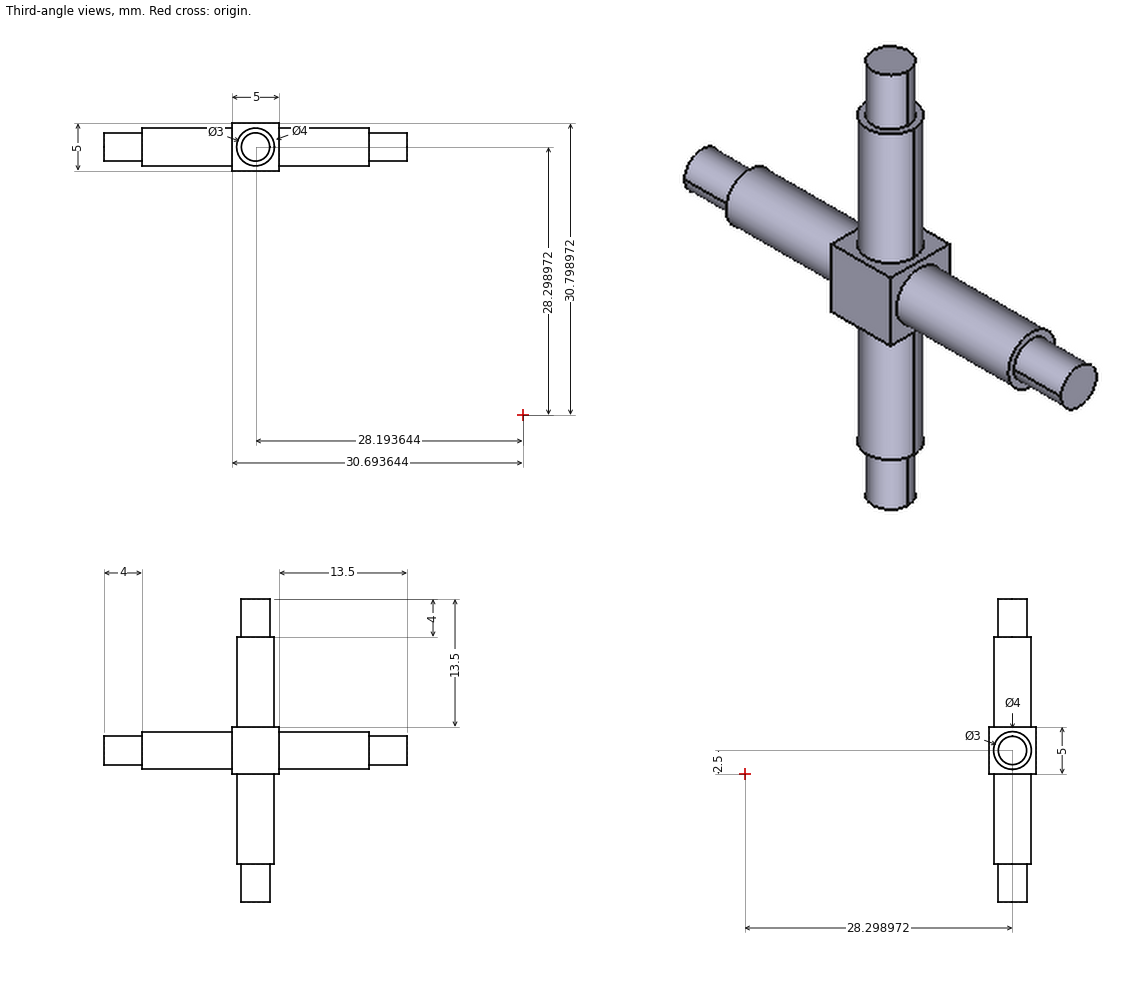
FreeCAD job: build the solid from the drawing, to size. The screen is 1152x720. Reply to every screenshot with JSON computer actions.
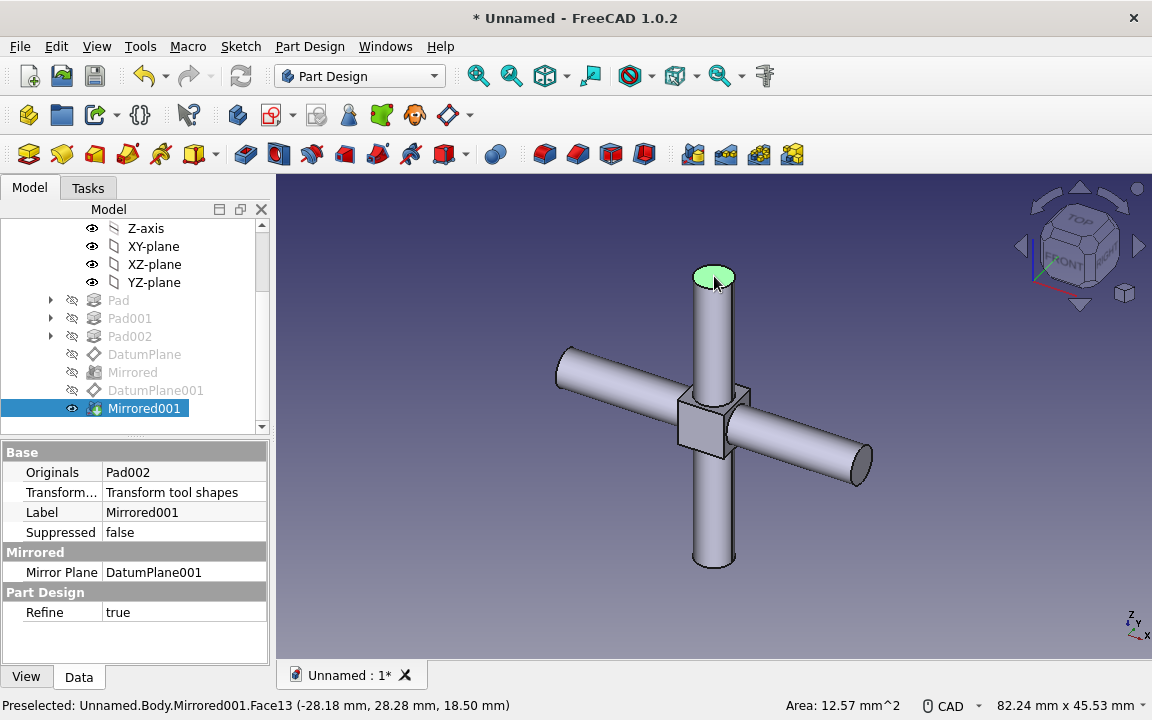
{"action": "left_click", "coordinate": [270, 116]}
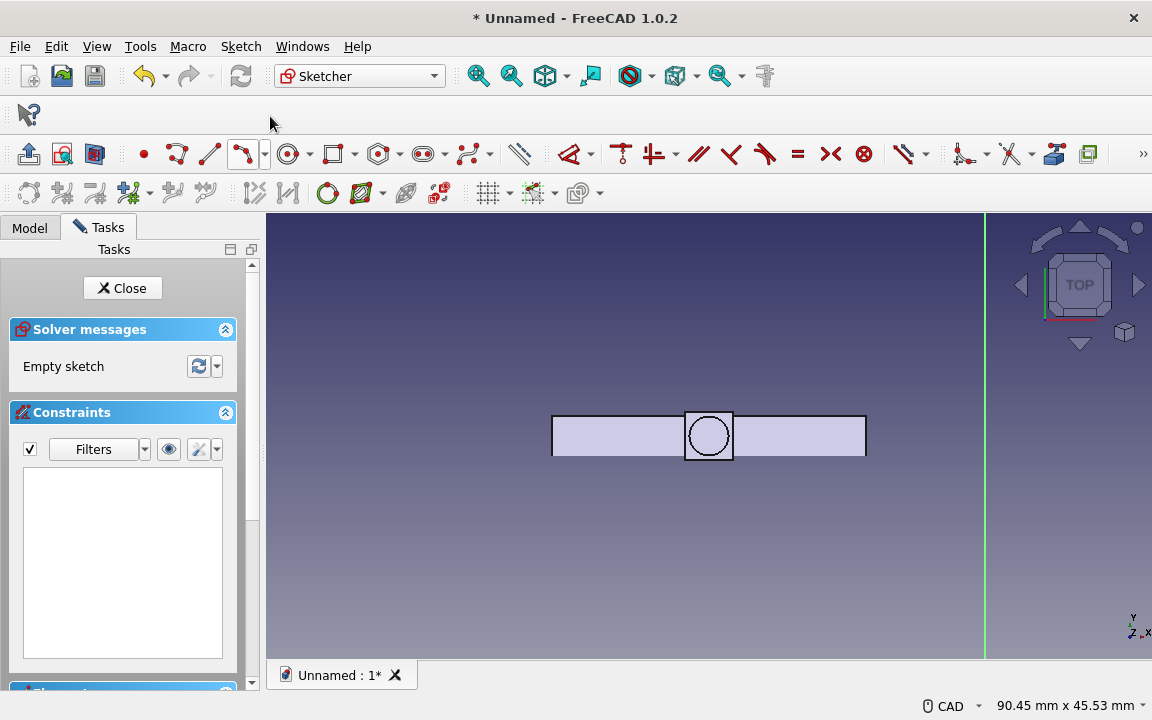
{"action": "scroll", "coordinate": [720, 436], "scroll_direction": "up", "scroll_amount": 10}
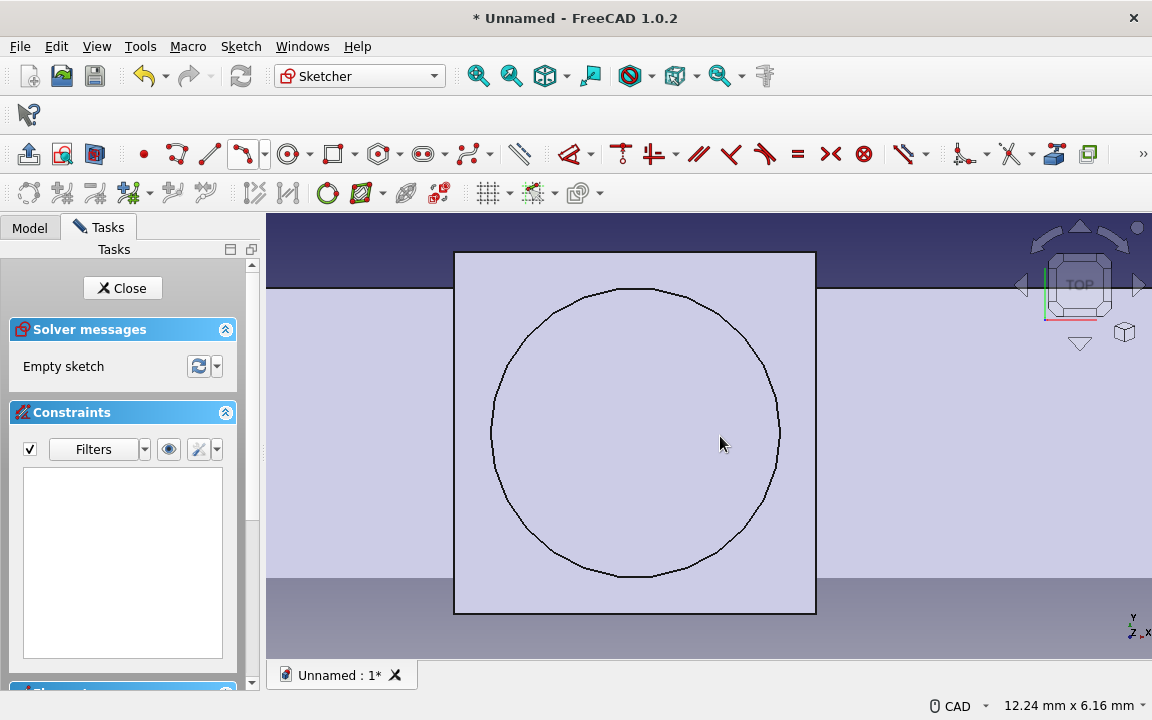
{"action": "key", "text": "g c"}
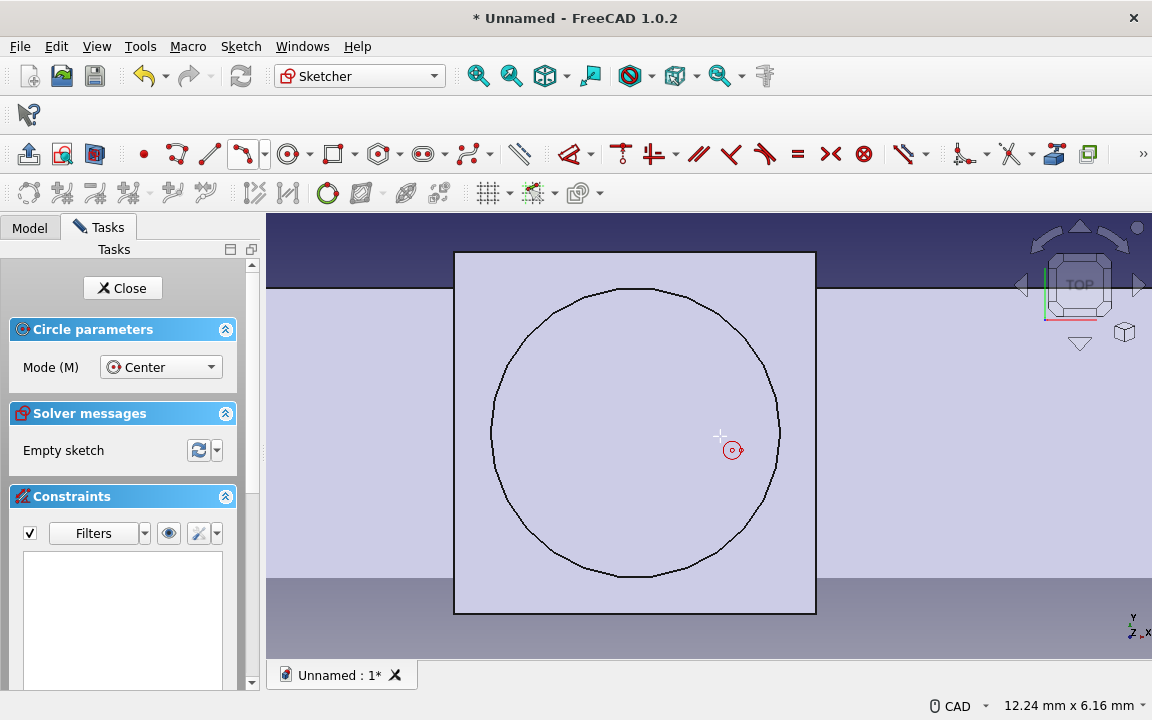
{"action": "left_click", "coordinate": [635, 433]}
{"action": "left_click", "coordinate": [738, 330]}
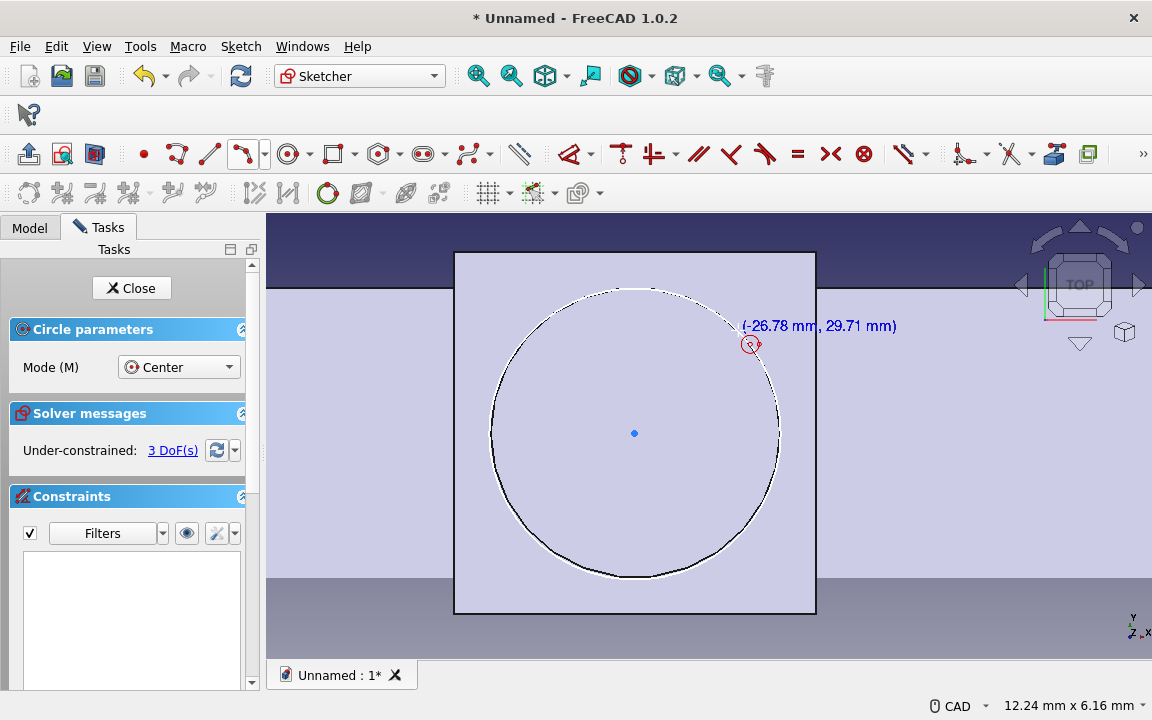
{"action": "left_click", "coordinate": [635, 434]}
{"action": "left_click", "coordinate": [712, 356]}
{"action": "key", "text": "Escape"}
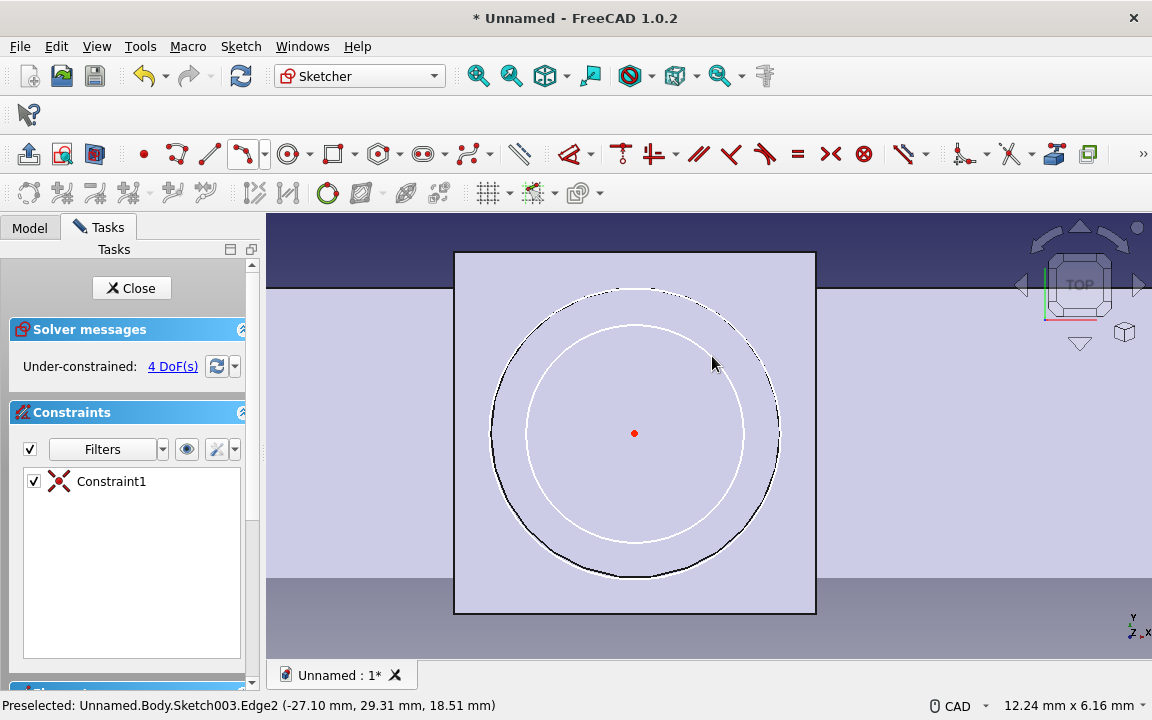
{"action": "left_click", "coordinate": [568, 154]}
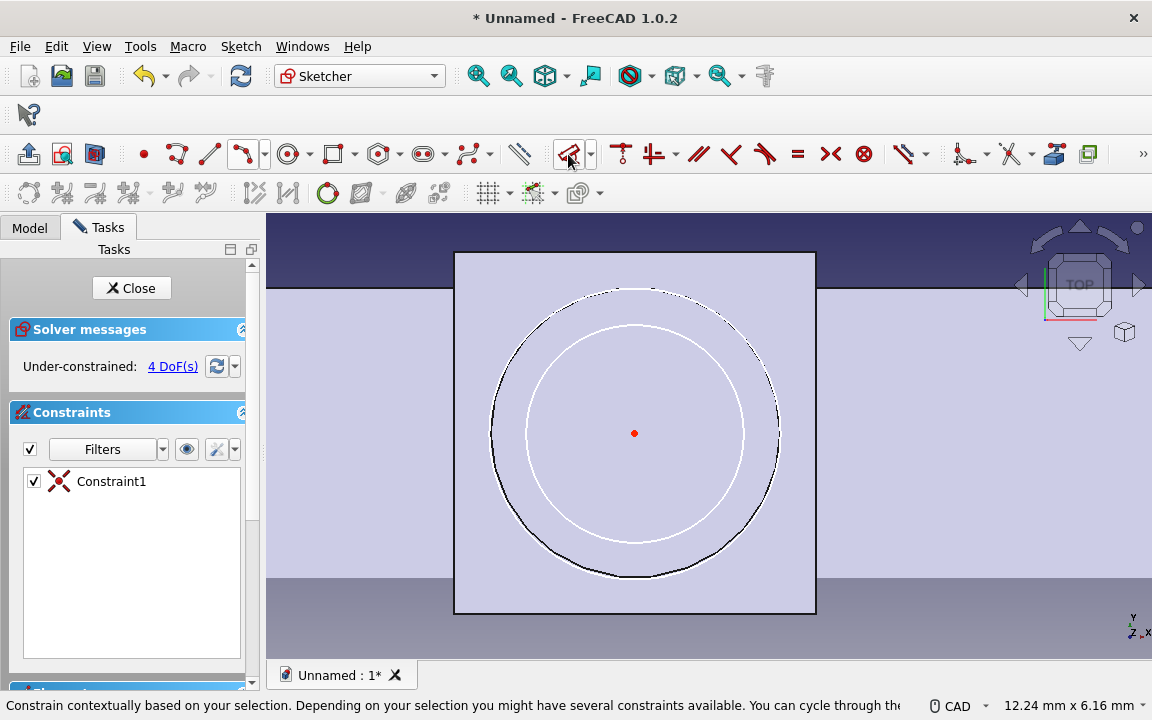
{"action": "left_click", "coordinate": [738, 331]}
{"action": "left_click", "coordinate": [761, 308]}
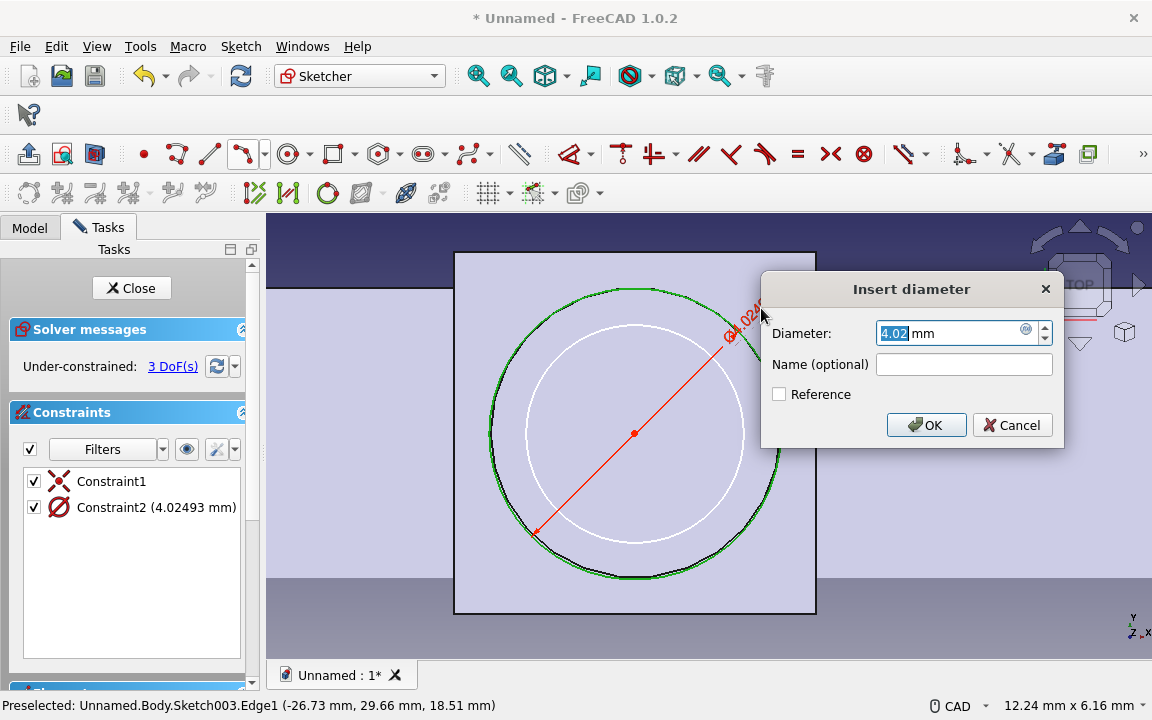
{"action": "type", "text": "4"}
{"action": "key", "text": "Return"}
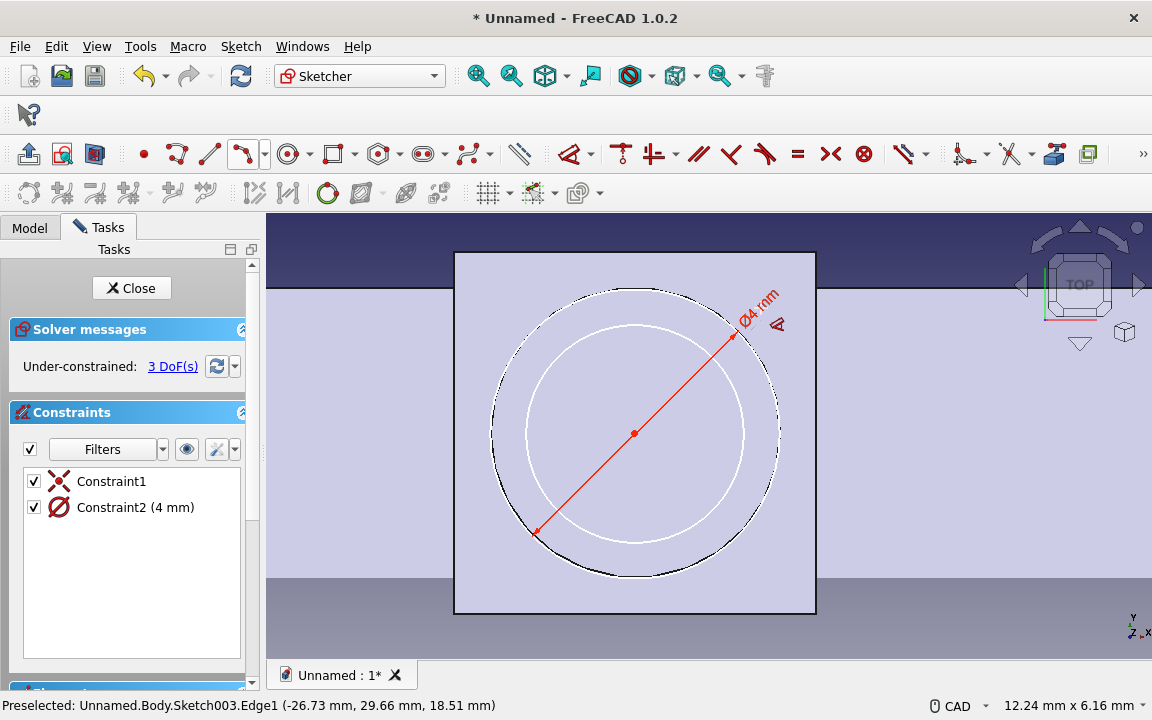
{"action": "left_click", "coordinate": [712, 357]}
{"action": "left_click", "coordinate": [792, 388]}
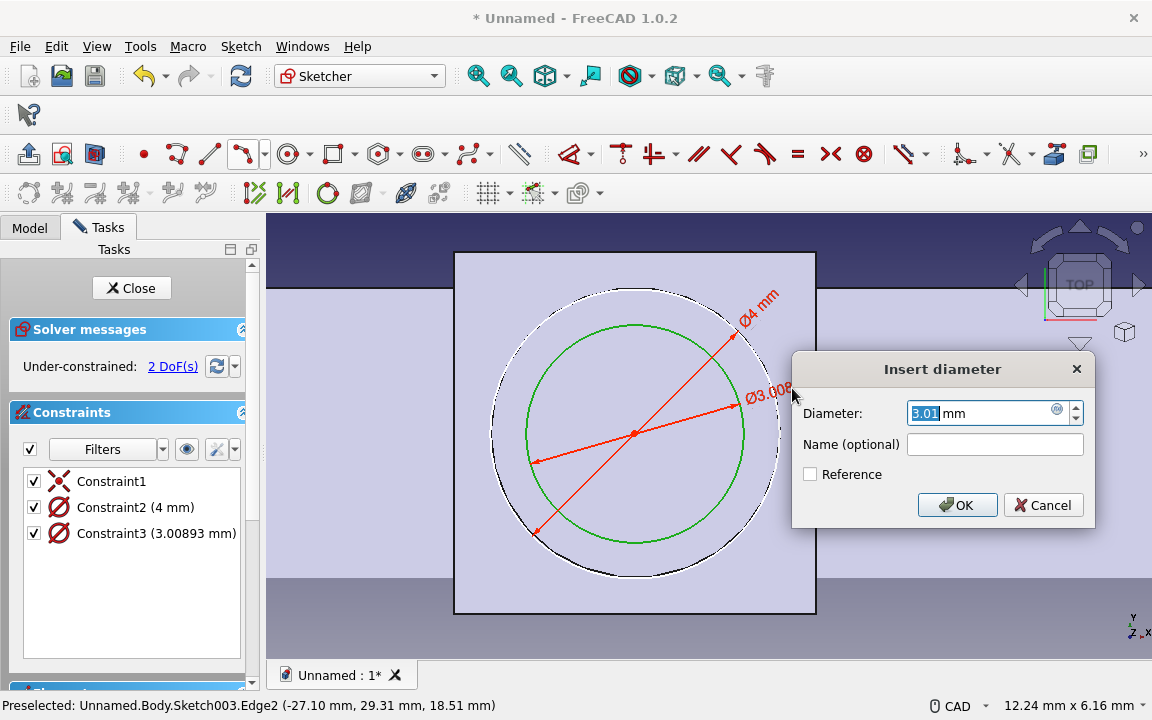
{"action": "type", "text": "3"}
{"action": "key", "text": "Return"}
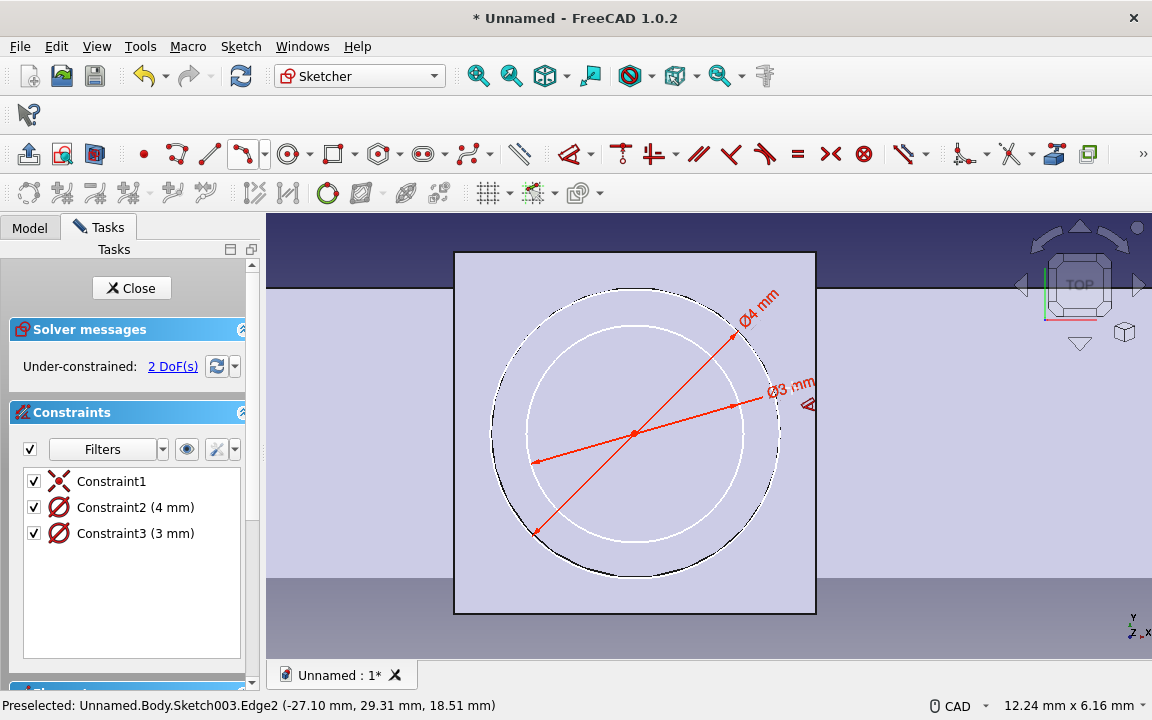
{"action": "left_click", "coordinate": [635, 434]}
{"action": "left_click", "coordinate": [892, 400]}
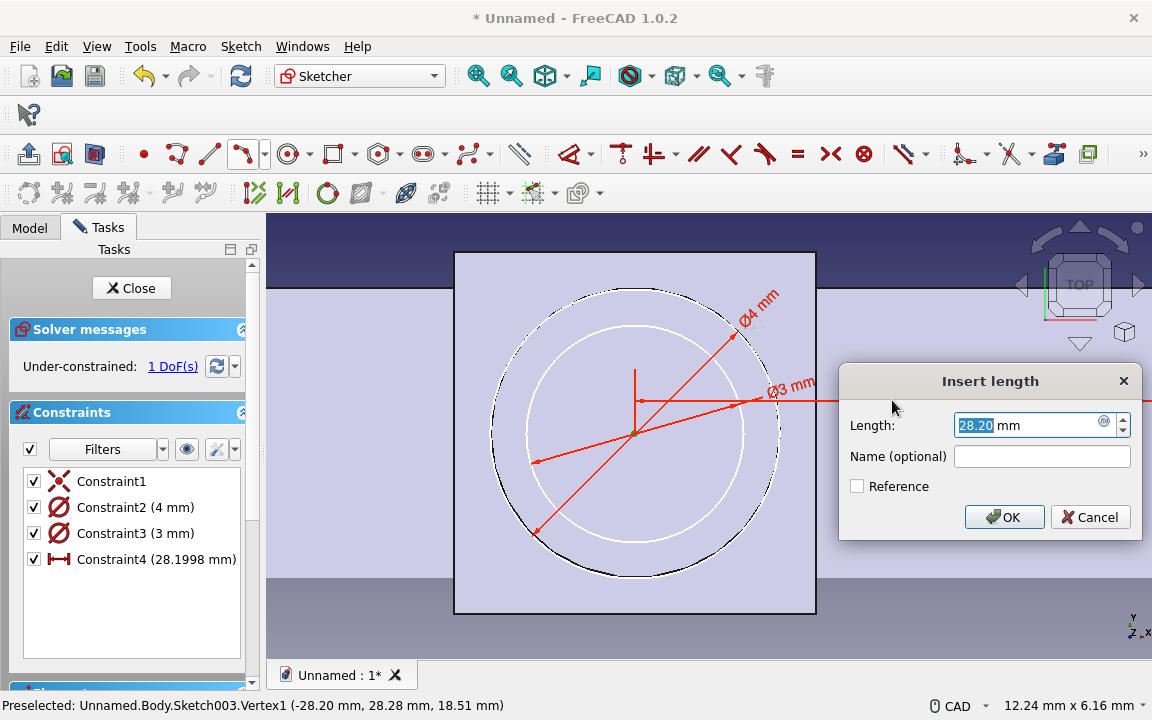
{"action": "type", "text": "28.193644"}
{"action": "key", "text": "Return"}